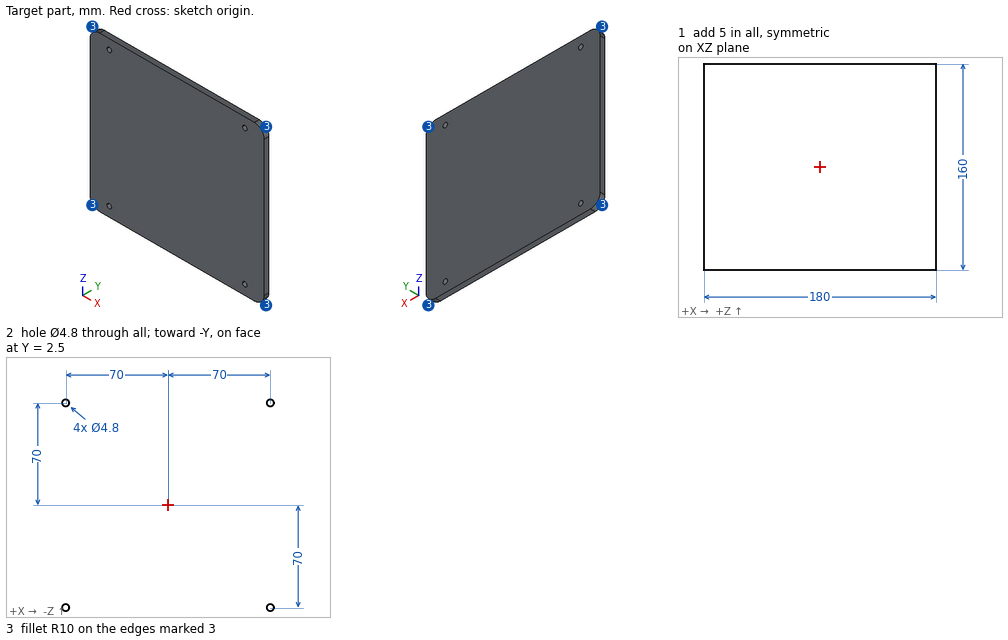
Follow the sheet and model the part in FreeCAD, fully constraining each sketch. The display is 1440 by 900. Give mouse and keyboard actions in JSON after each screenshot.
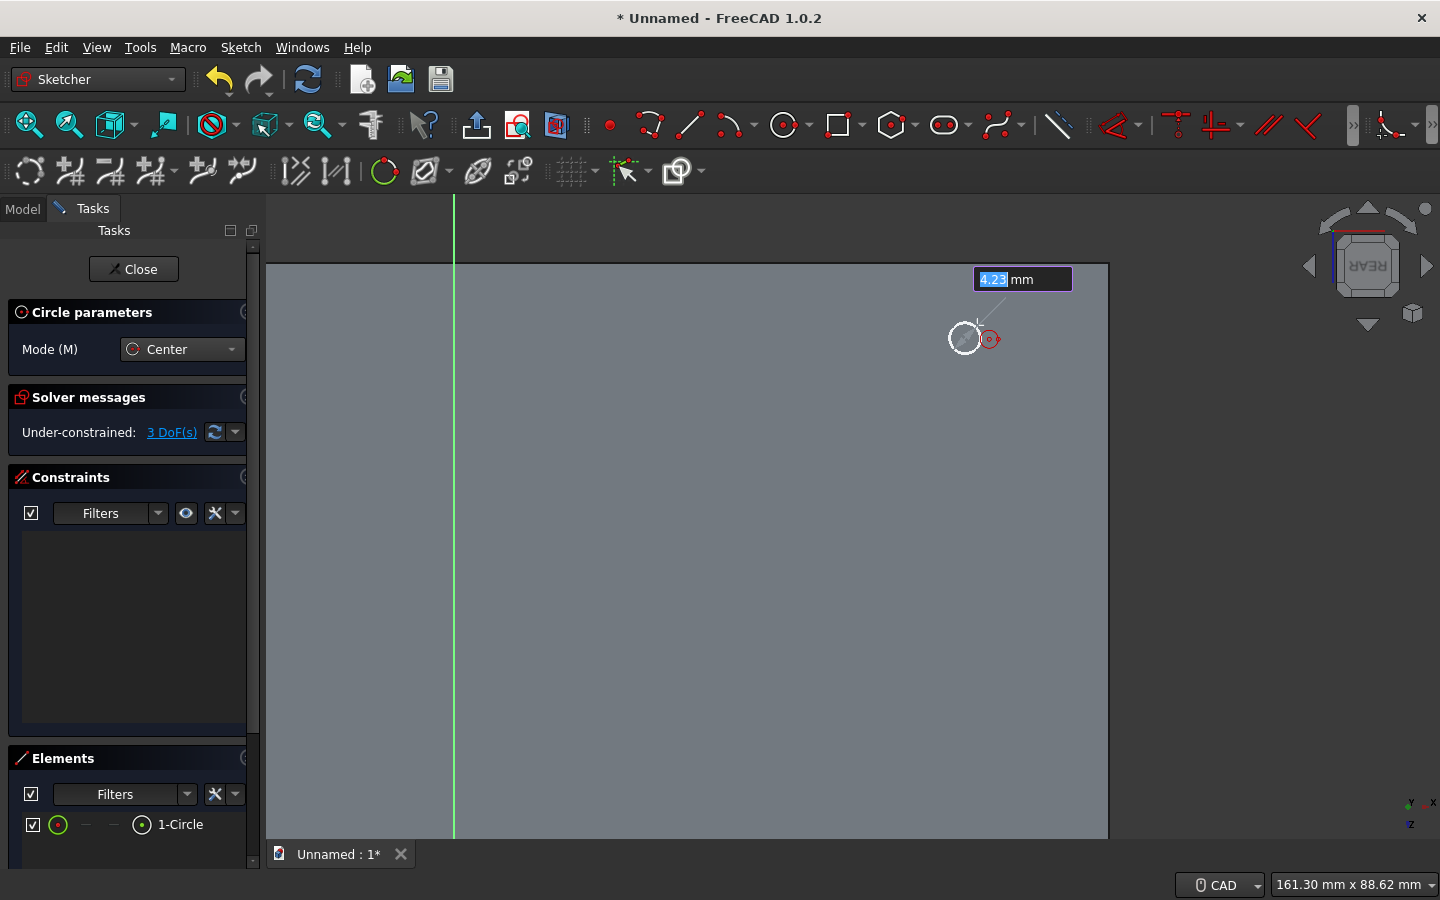
{"action": "left_click", "coordinate": [976, 323]}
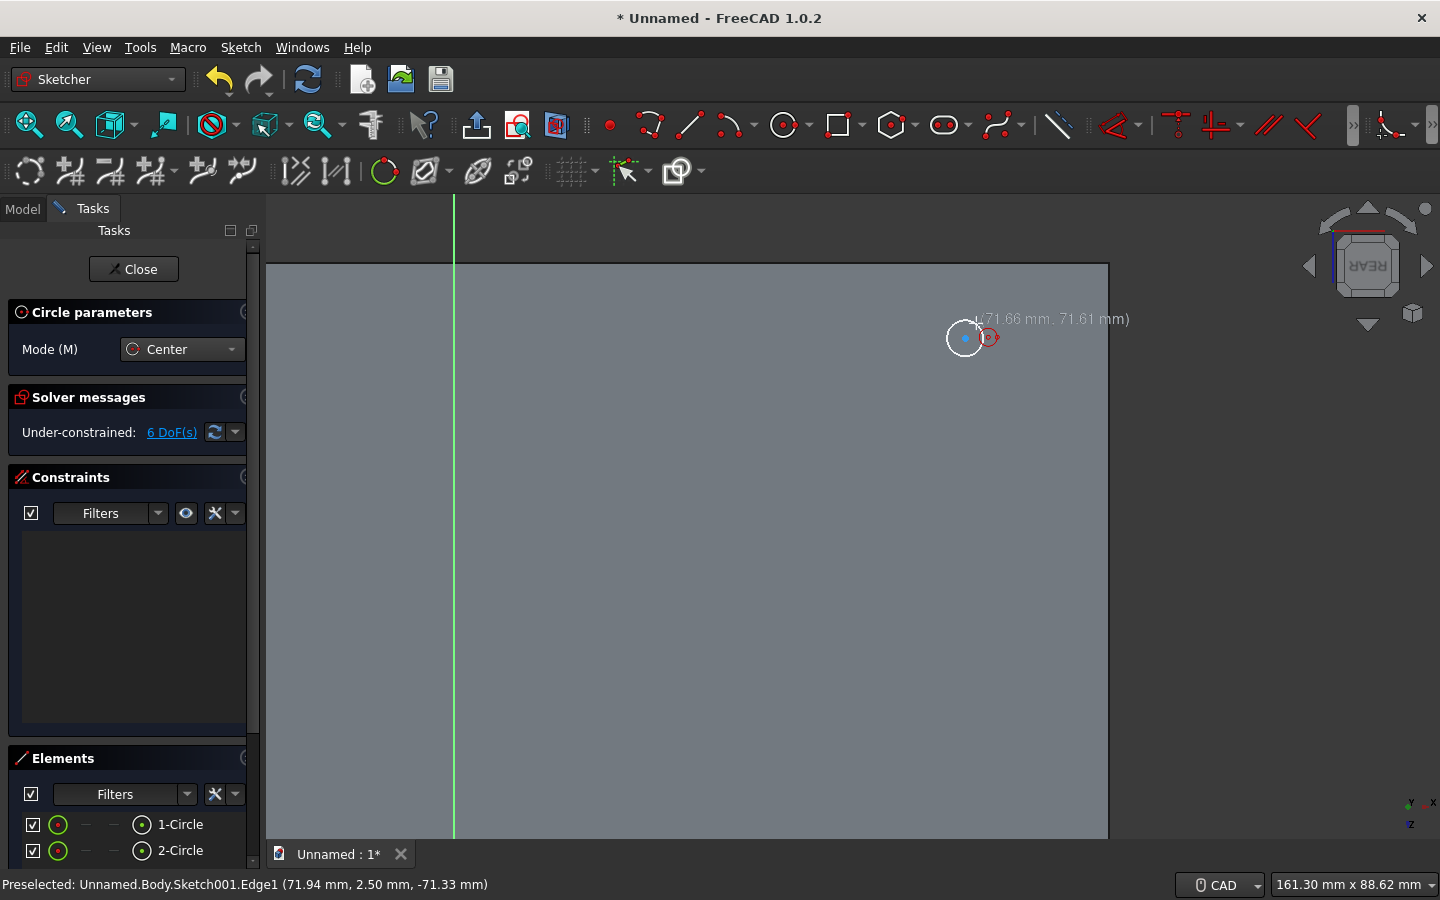
{"action": "scroll", "coordinate": [977, 325], "scroll_direction": "down", "scroll_amount": 5}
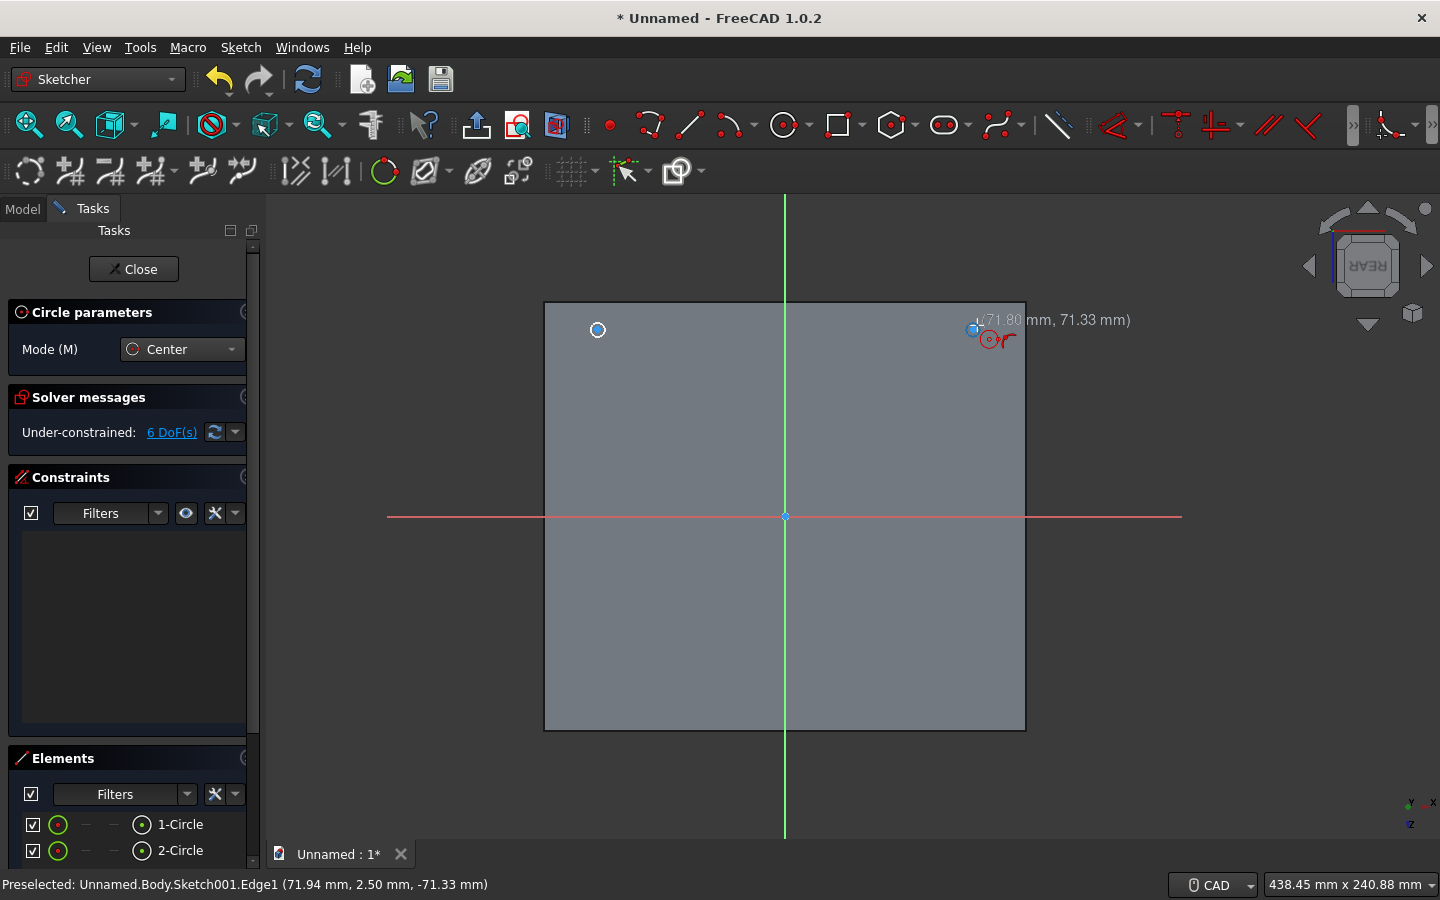
{"action": "scroll", "coordinate": [973, 704], "scroll_direction": "up", "scroll_amount": 7}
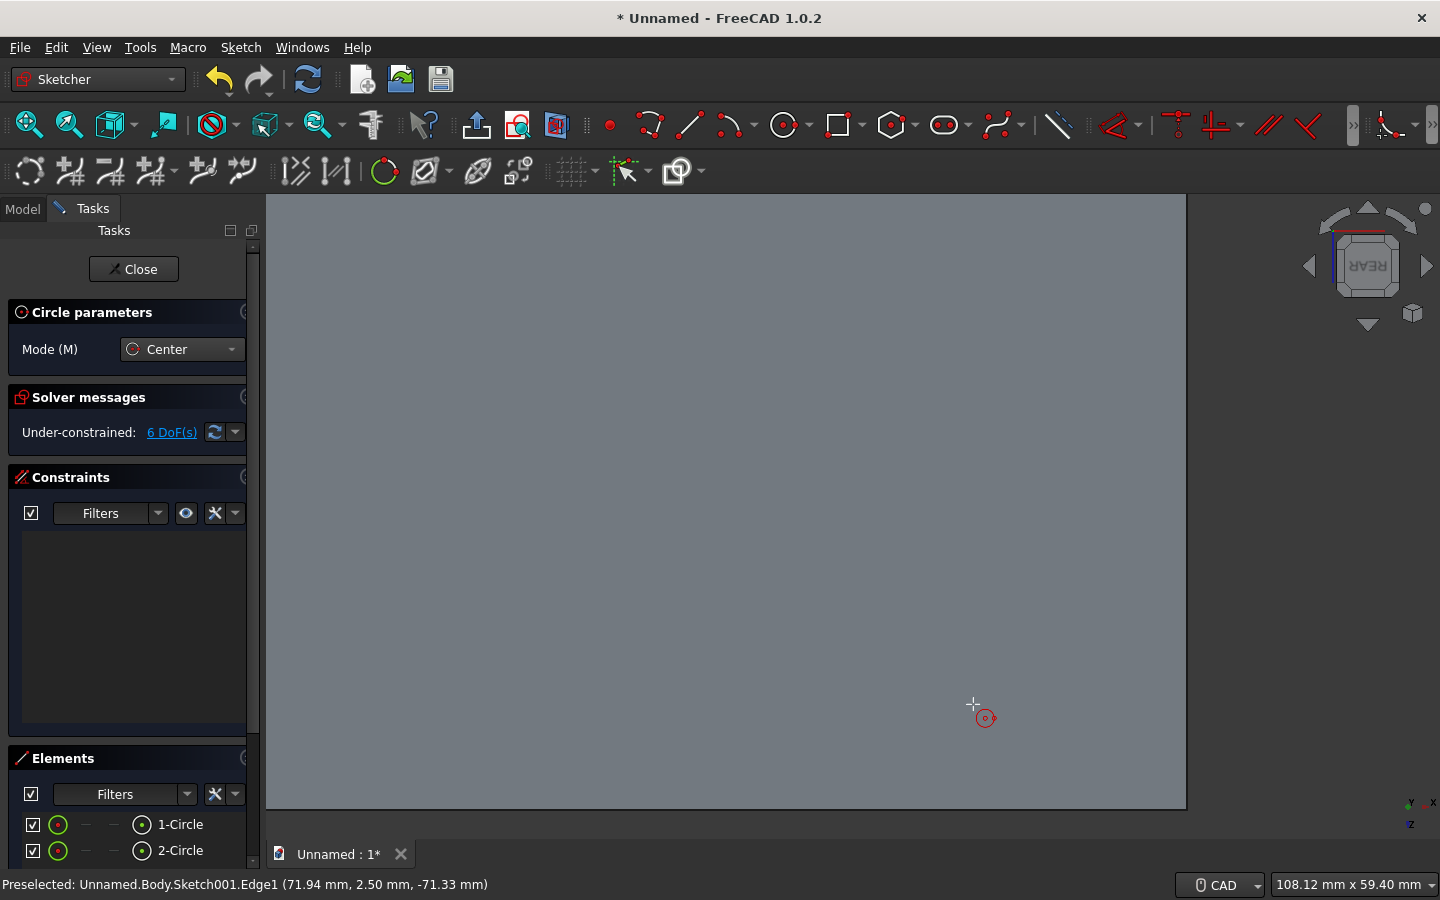
{"action": "scroll", "coordinate": [973, 705], "scroll_direction": "down", "scroll_amount": 7}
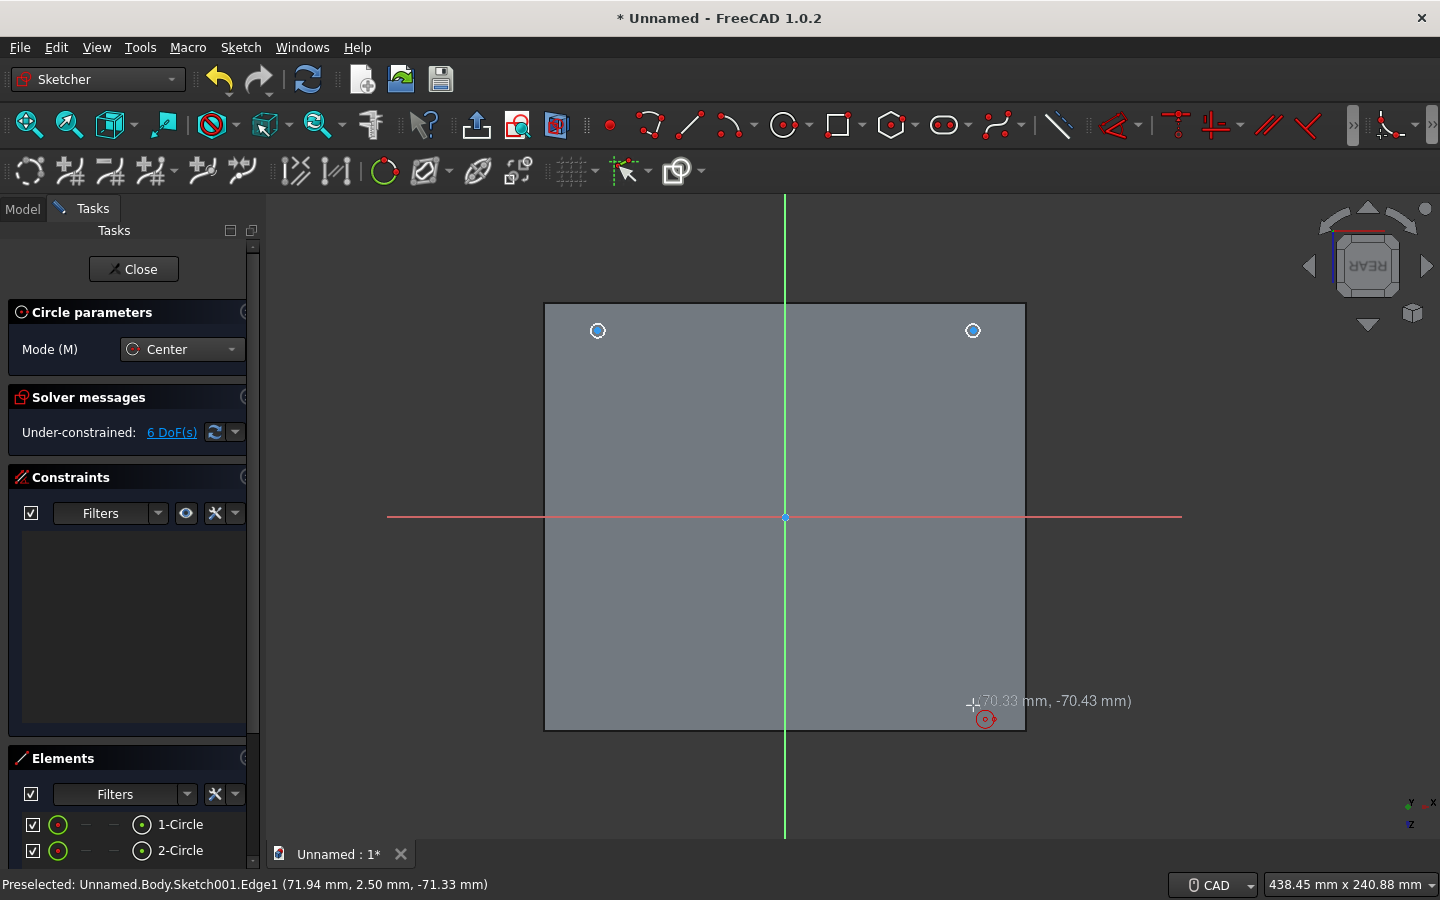
{"action": "left_click", "coordinate": [973, 705]}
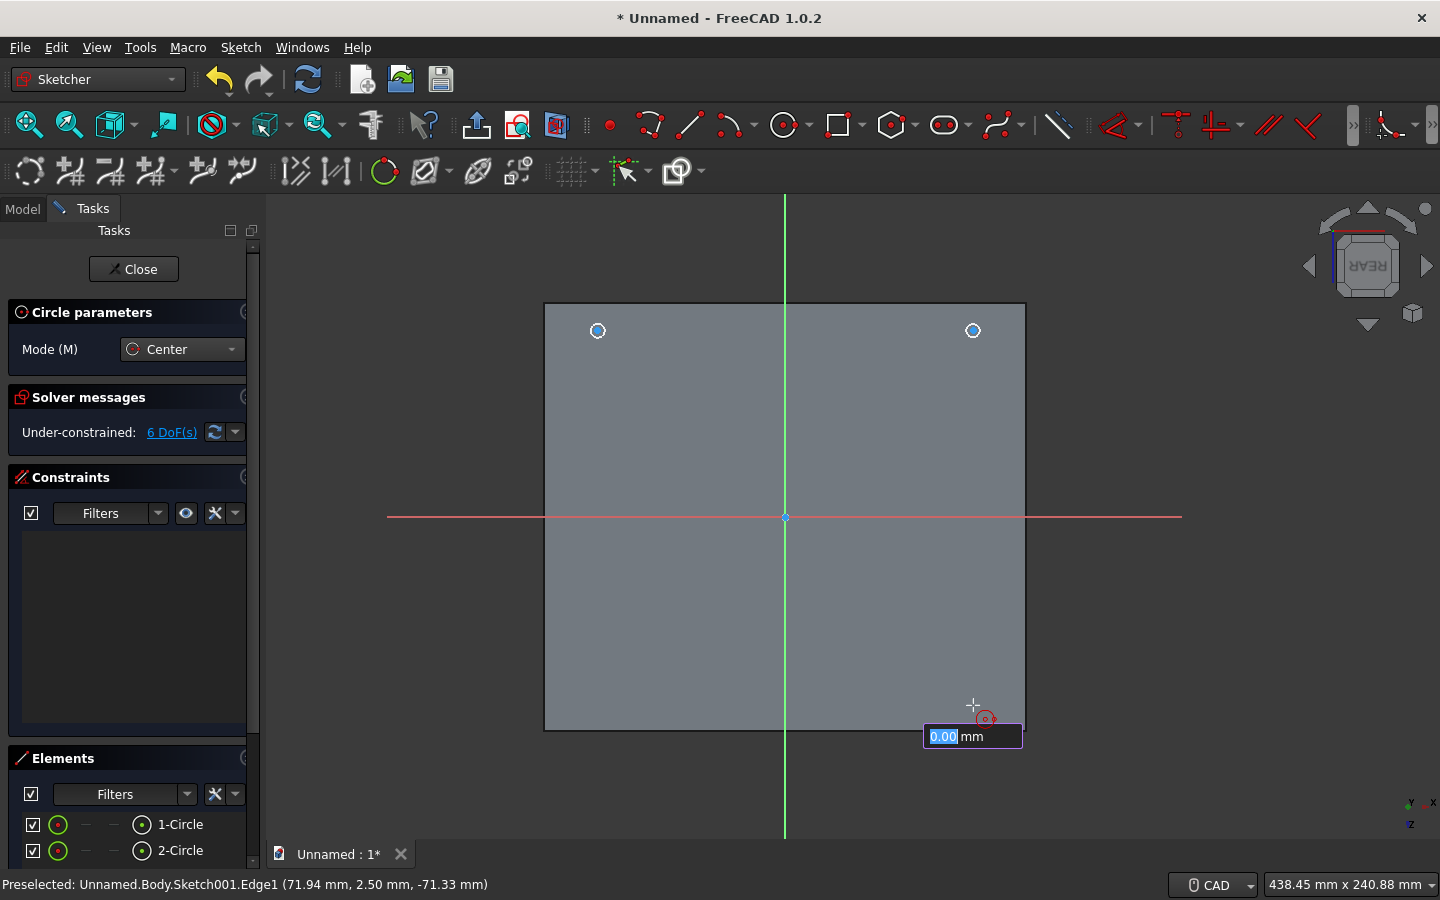
{"action": "scroll", "coordinate": [977, 700], "scroll_direction": "up", "scroll_amount": 5}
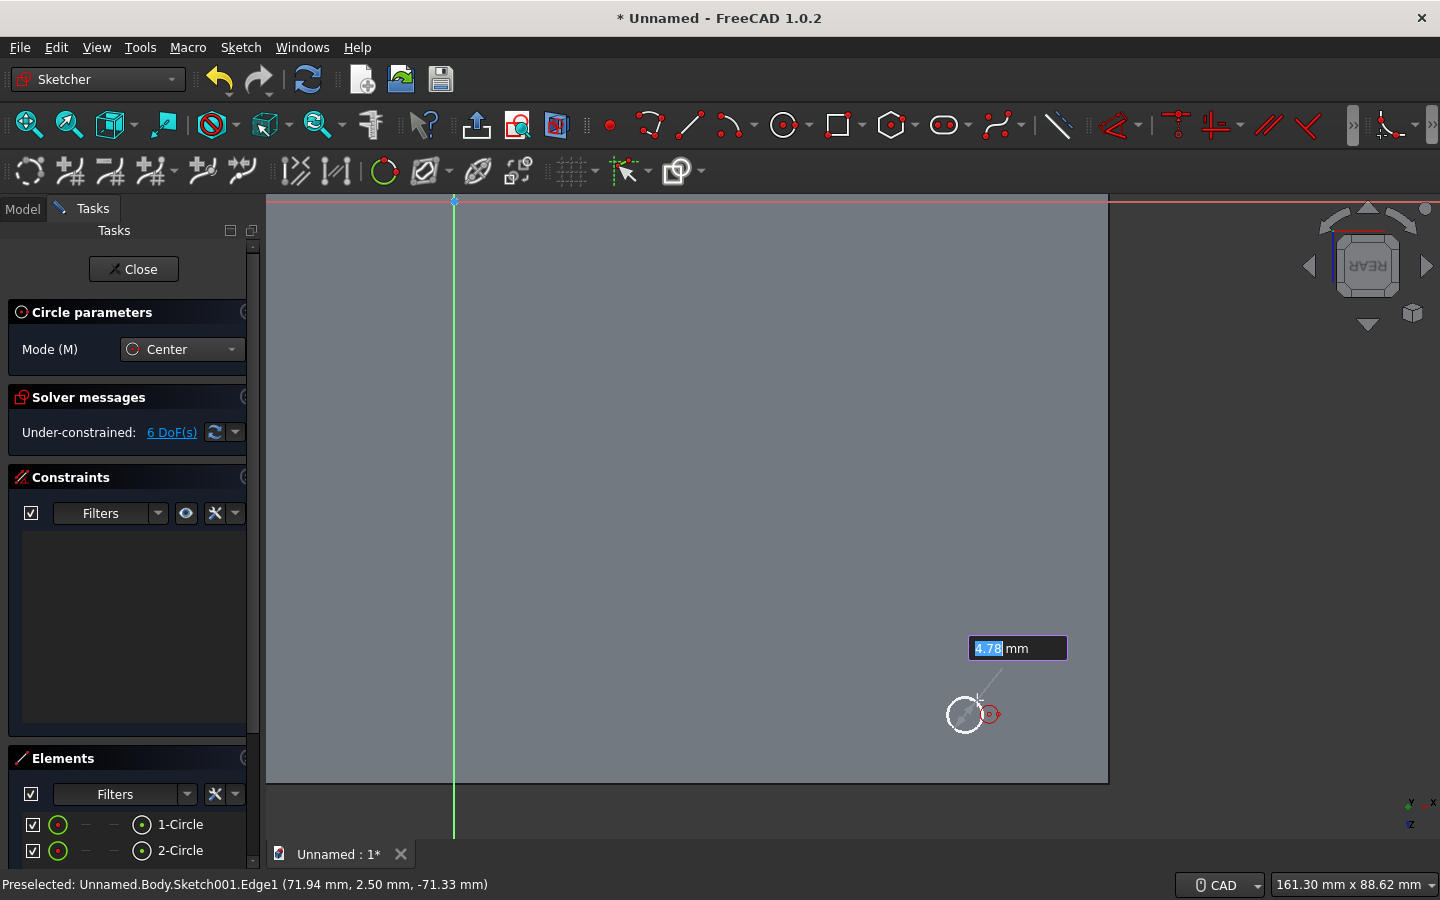
{"action": "left_click", "coordinate": [976, 699]}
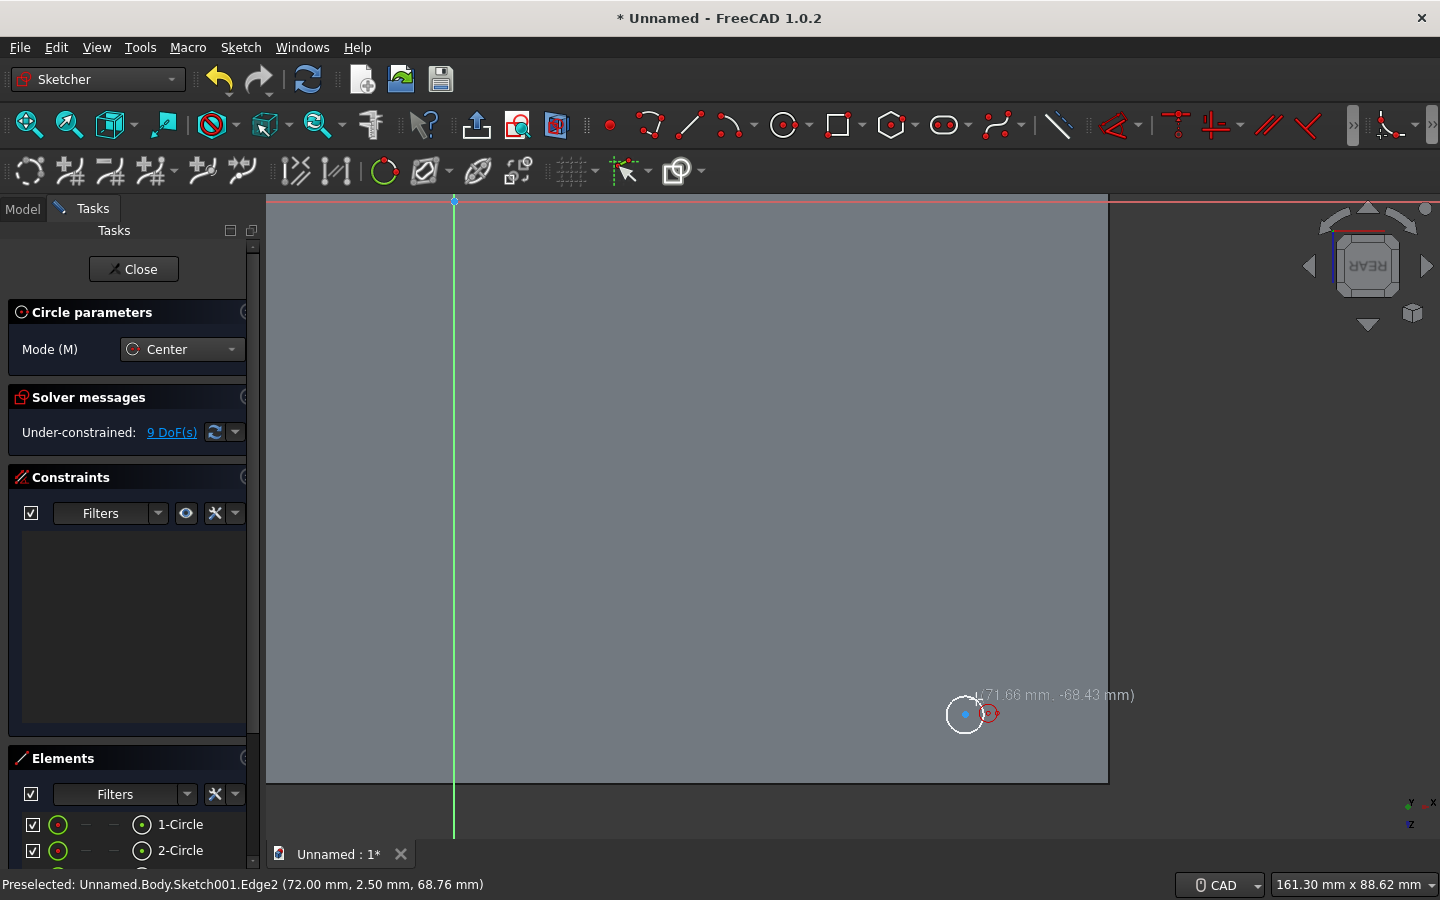
{"action": "scroll", "coordinate": [977, 700], "scroll_direction": "down", "scroll_amount": 5}